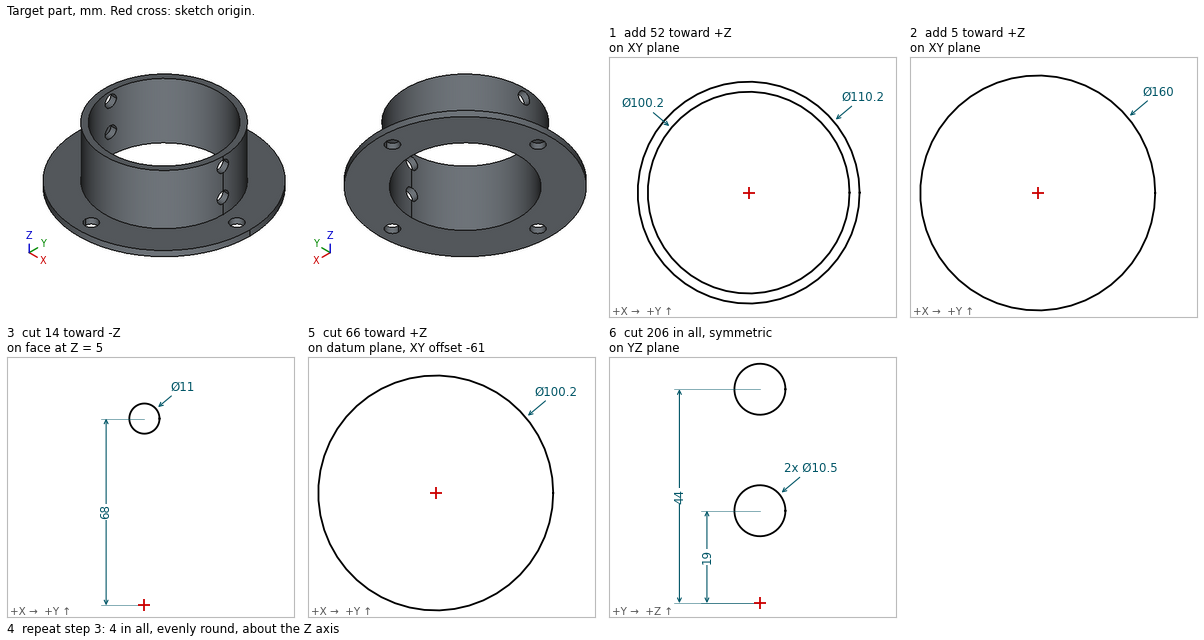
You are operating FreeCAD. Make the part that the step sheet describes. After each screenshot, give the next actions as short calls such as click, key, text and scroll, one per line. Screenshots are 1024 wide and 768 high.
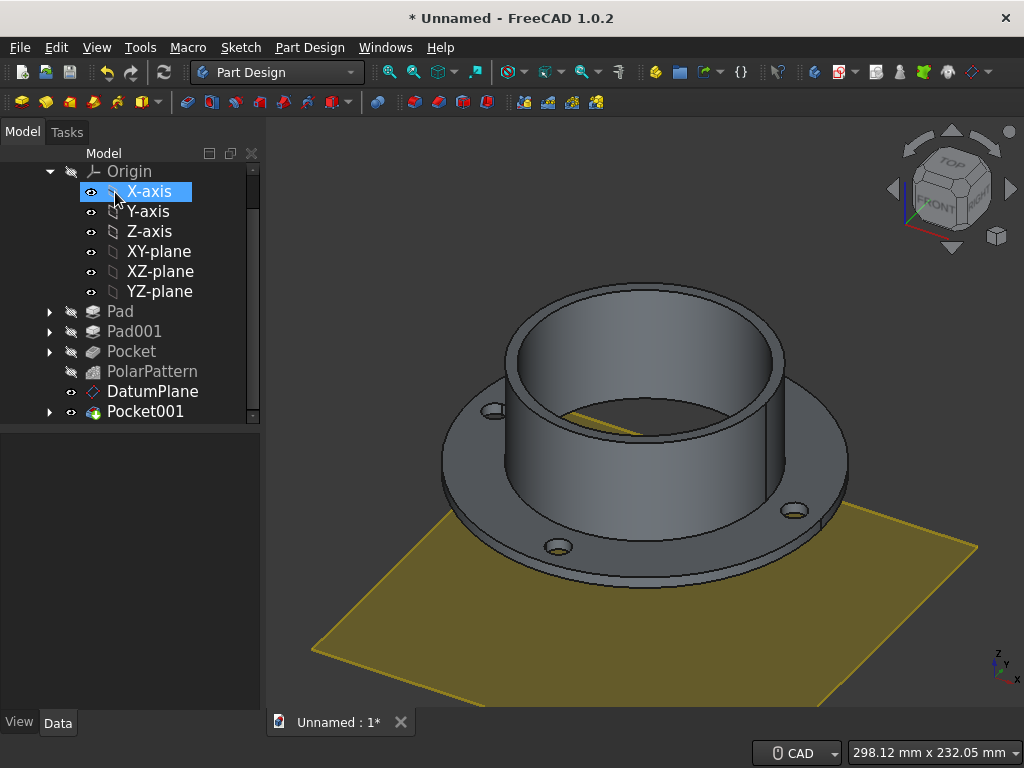
click(116, 392)
key(space)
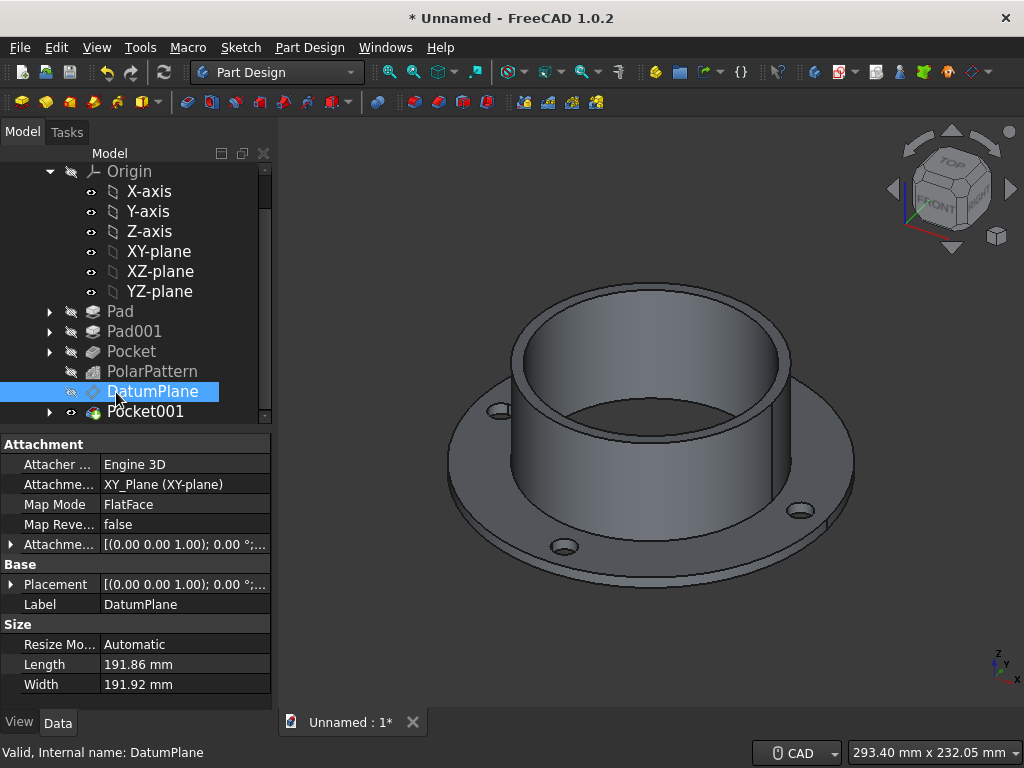
click(318, 667)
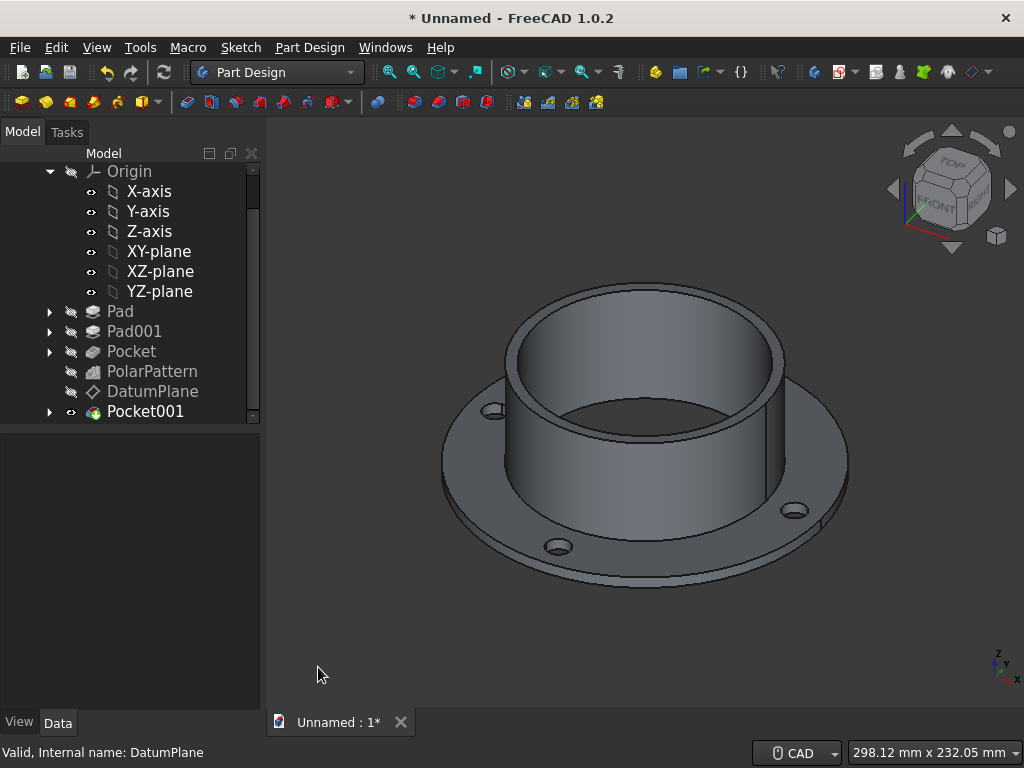
click(840, 72)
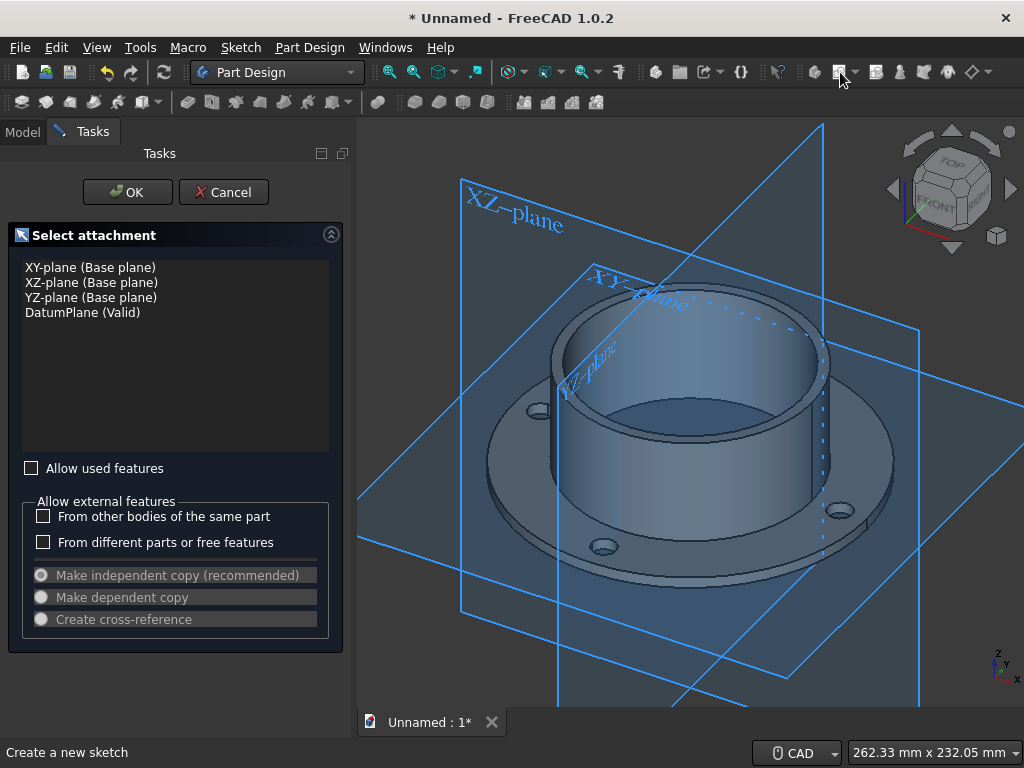
click(82, 298)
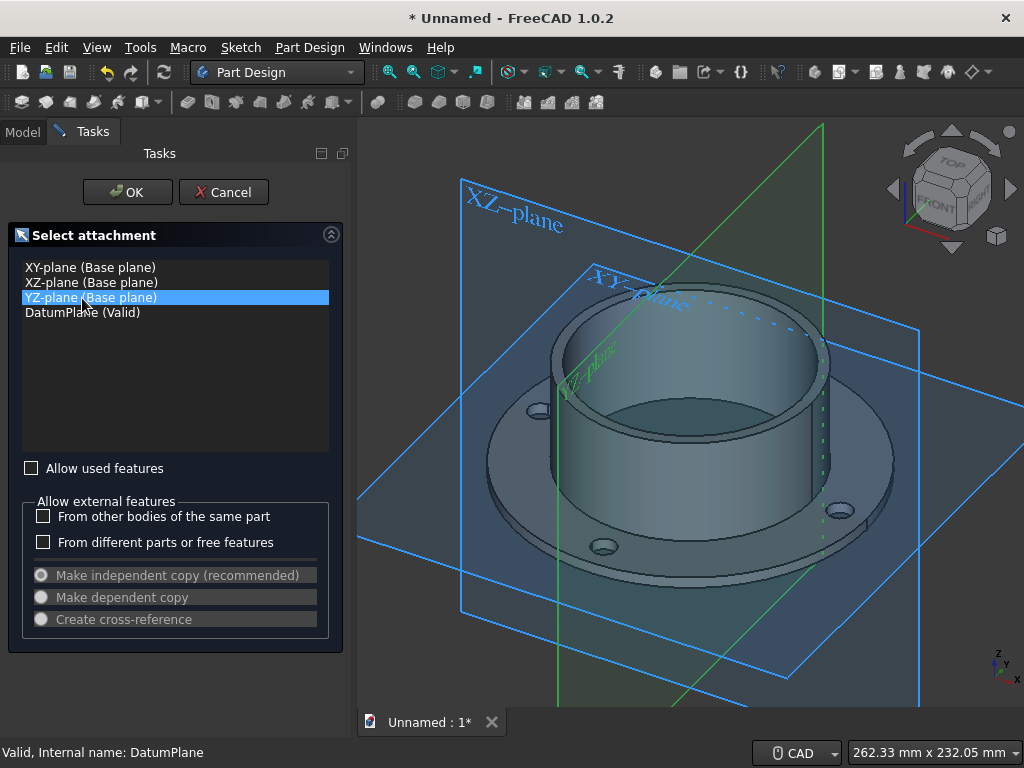
click(128, 192)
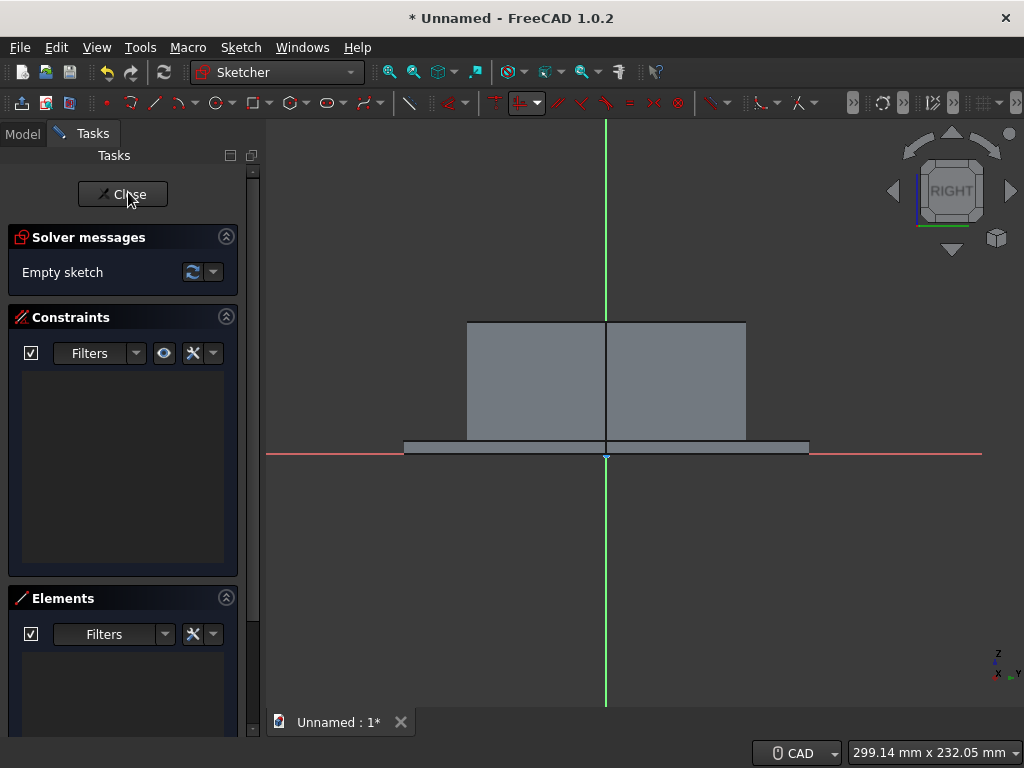
click(70, 104)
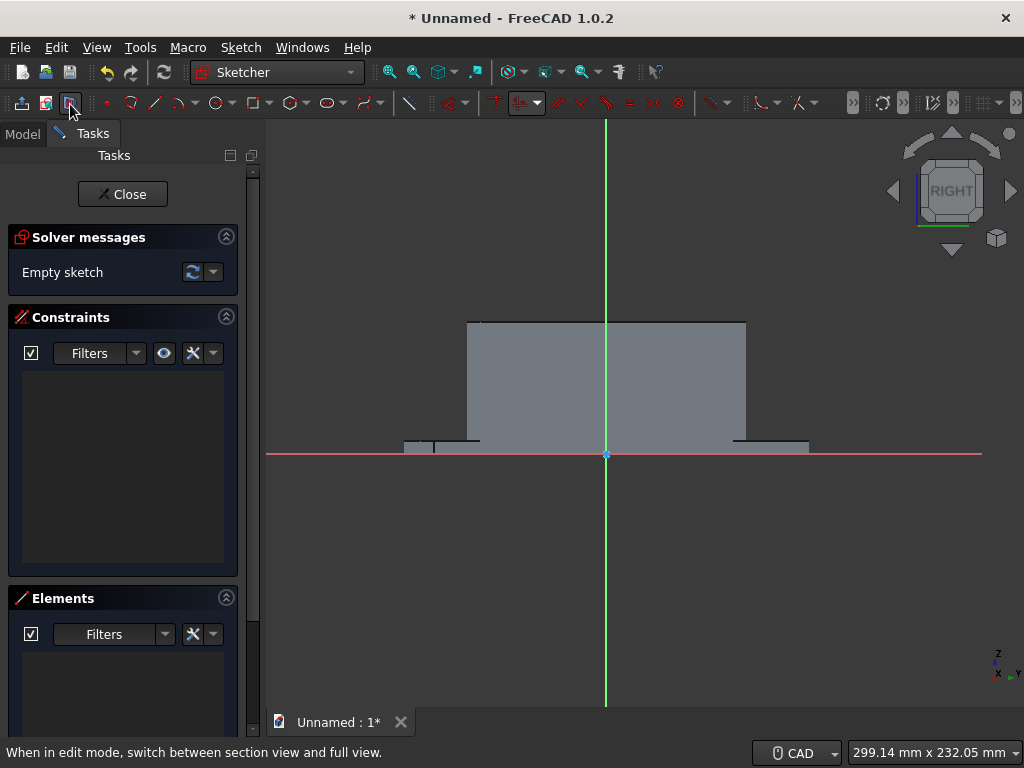
scroll(619, 382, up, 6)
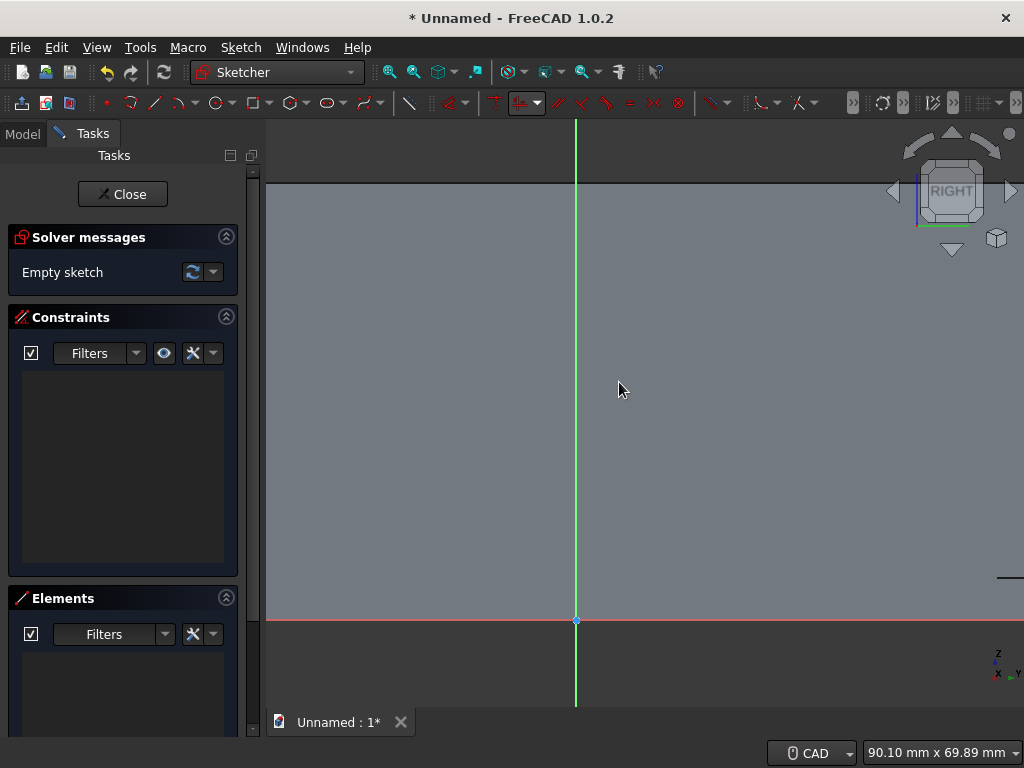
click(216, 104)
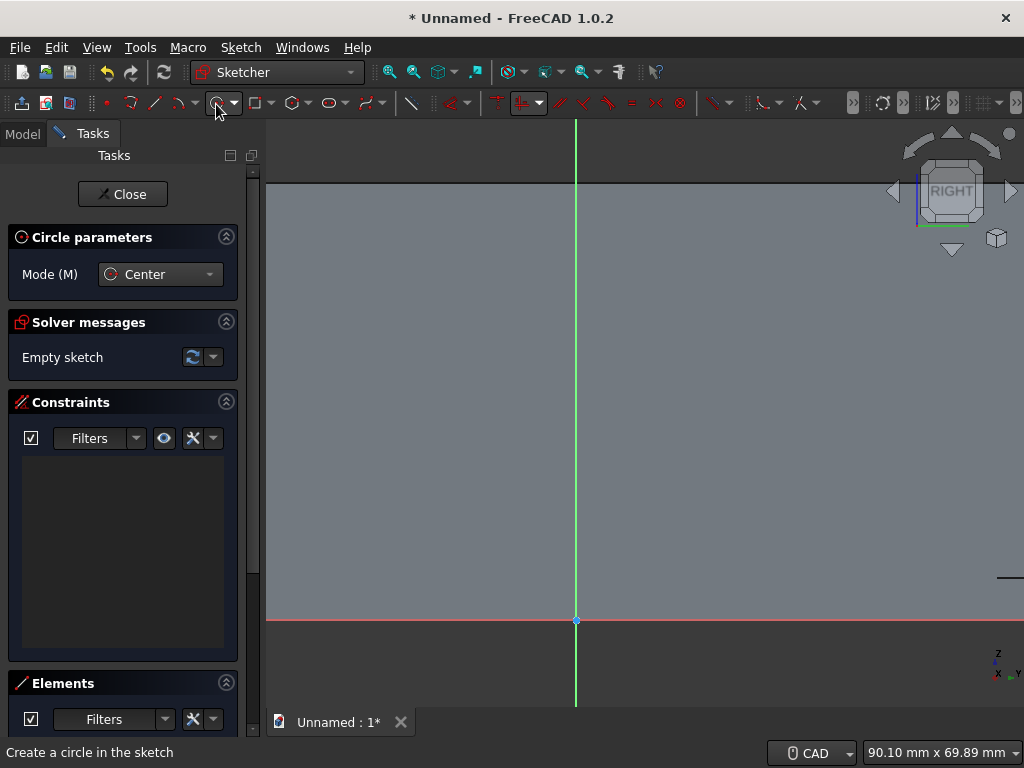
click(576, 460)
click(608, 429)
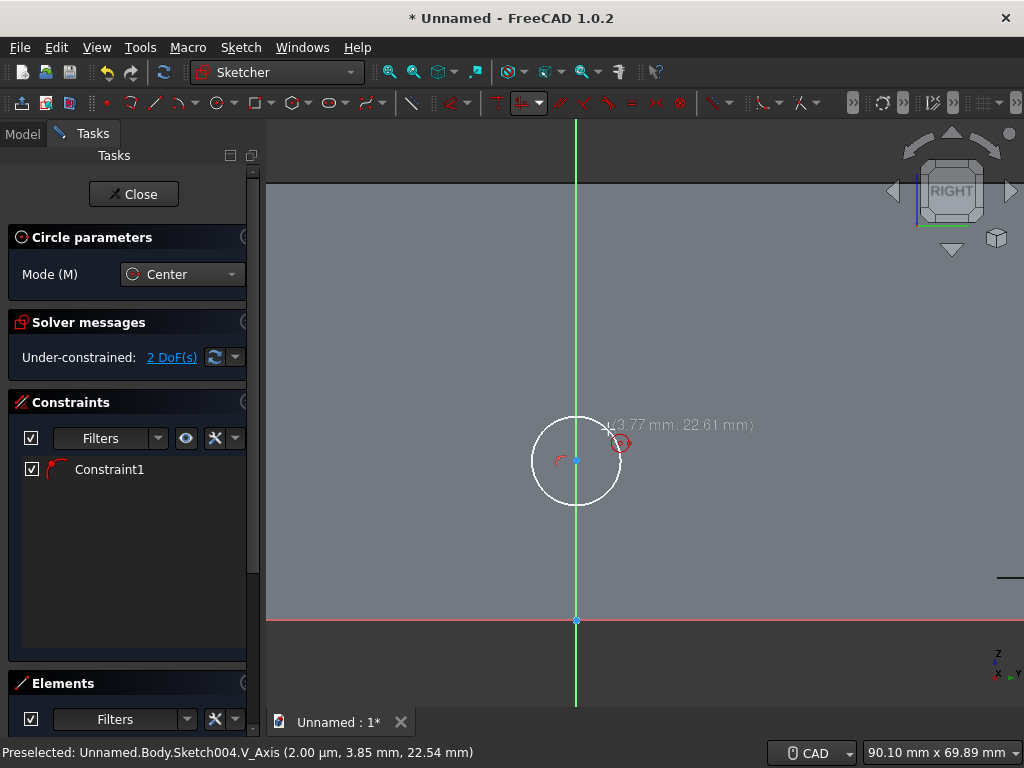
click(576, 250)
click(608, 219)
key(Escape)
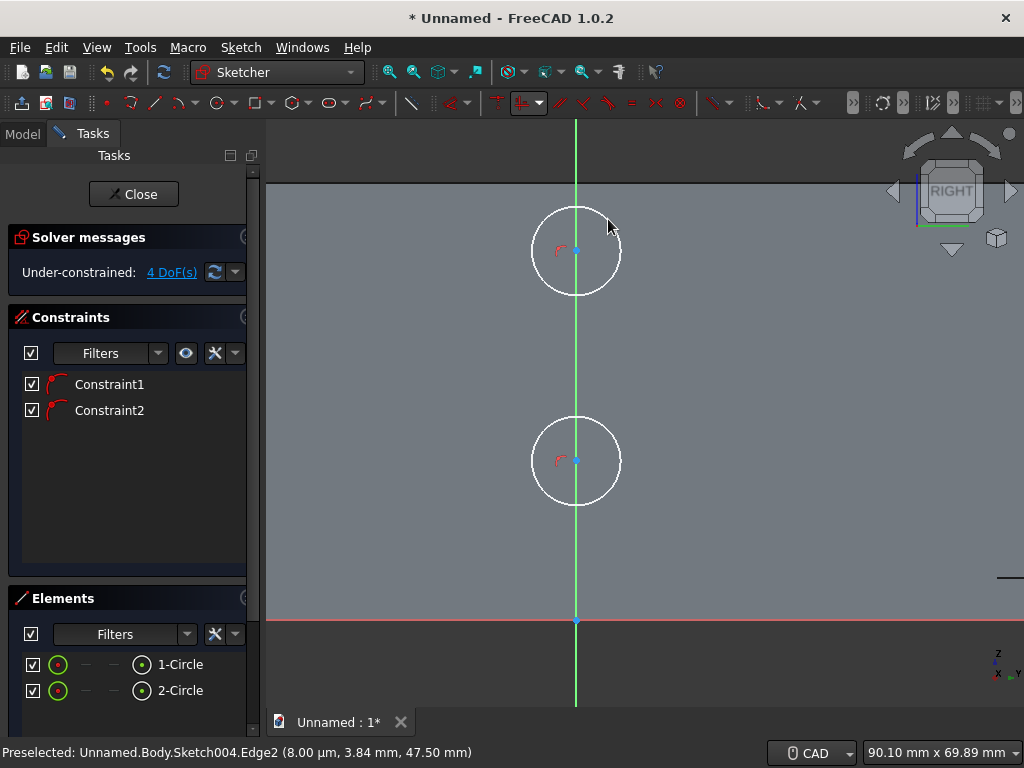
click(608, 430)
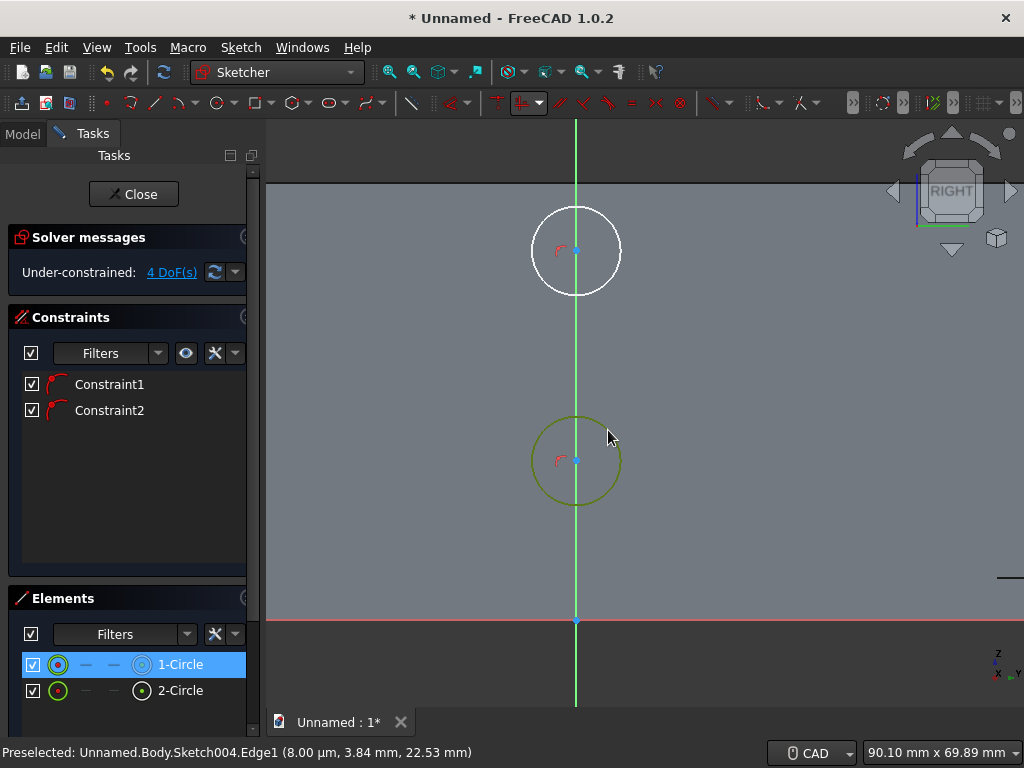
click(608, 220)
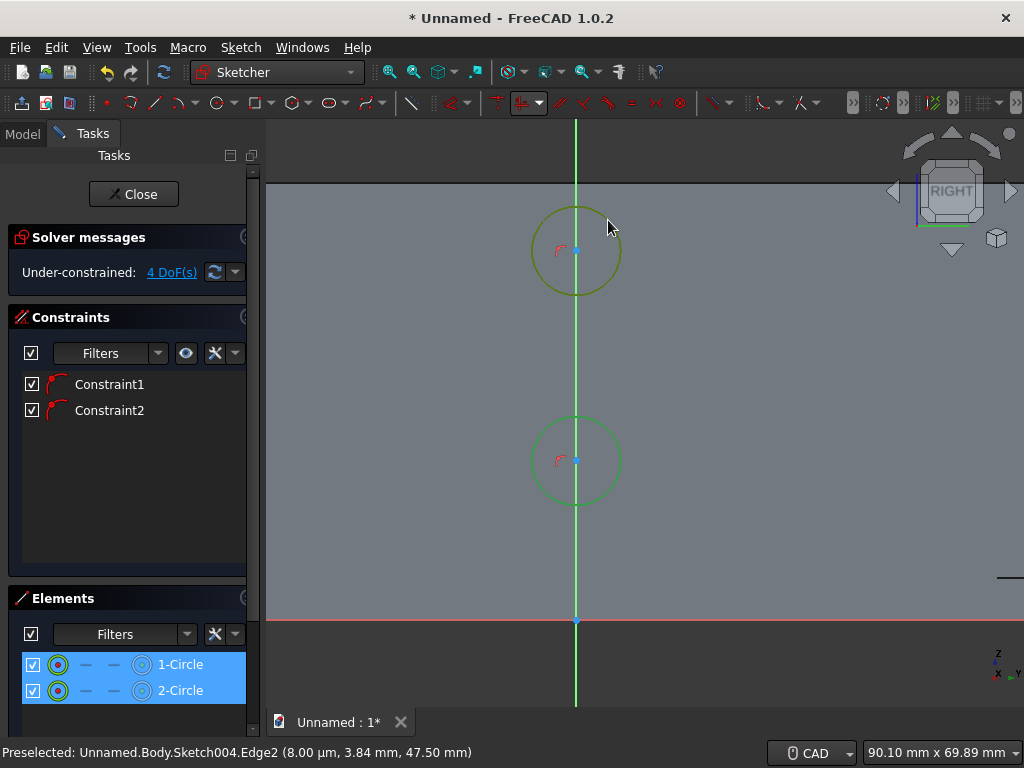
click(632, 104)